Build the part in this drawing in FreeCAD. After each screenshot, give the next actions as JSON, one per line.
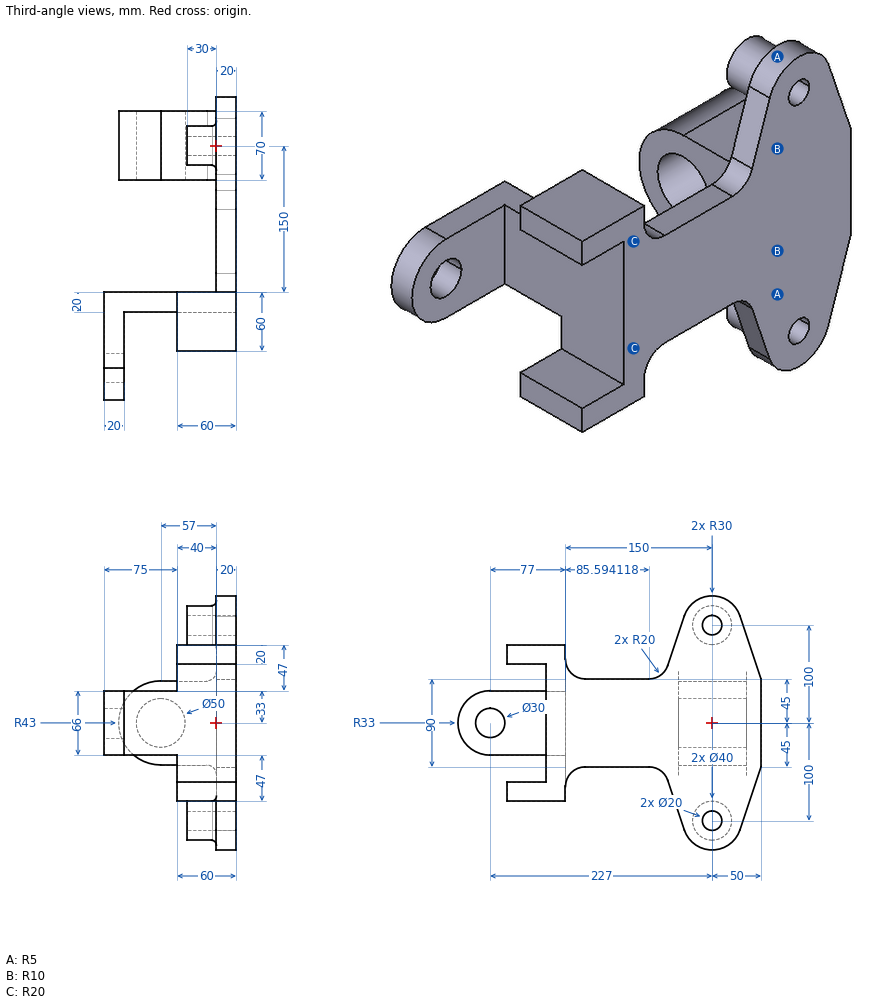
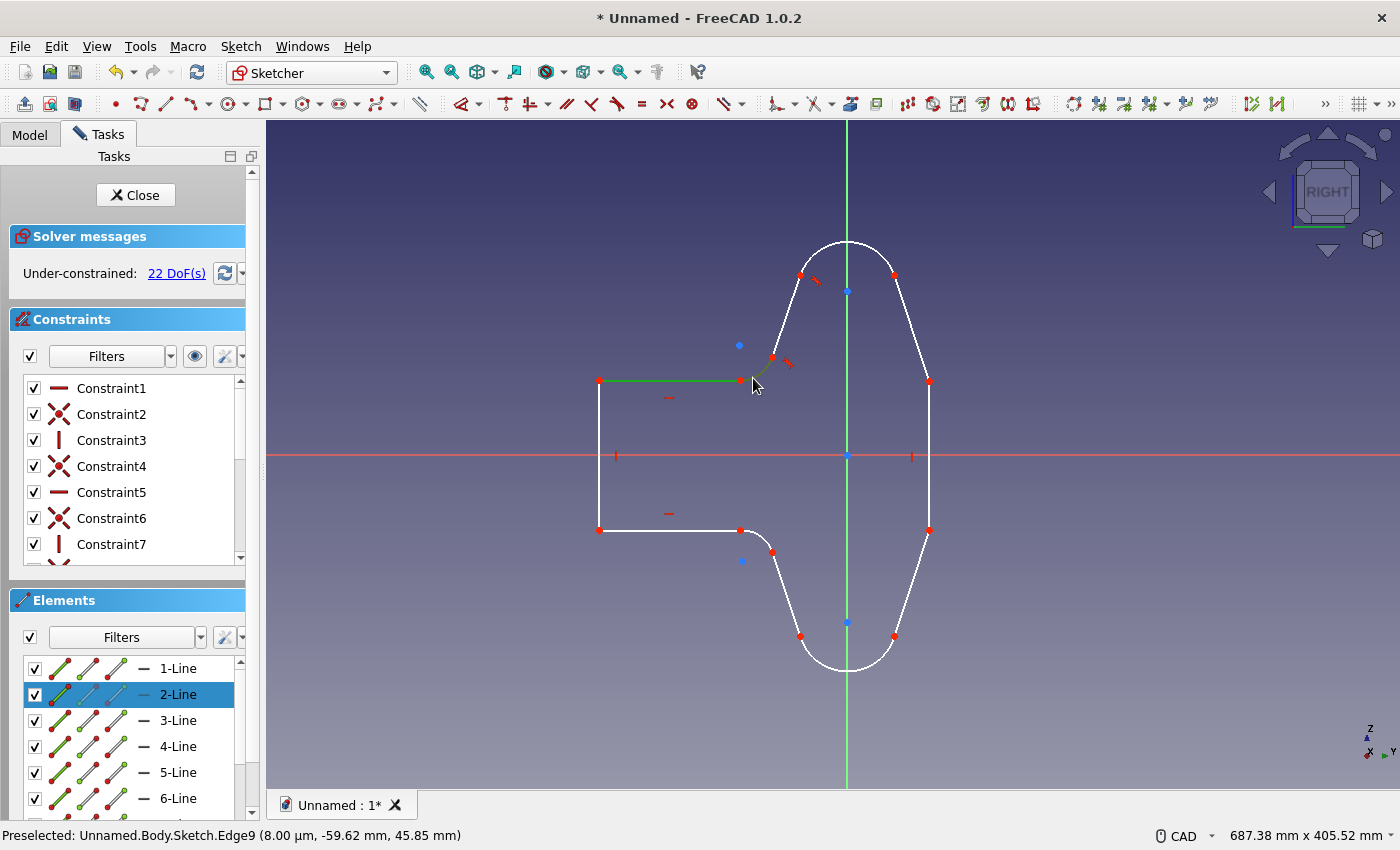
{"action": "left_click", "coordinate": [617, 104]}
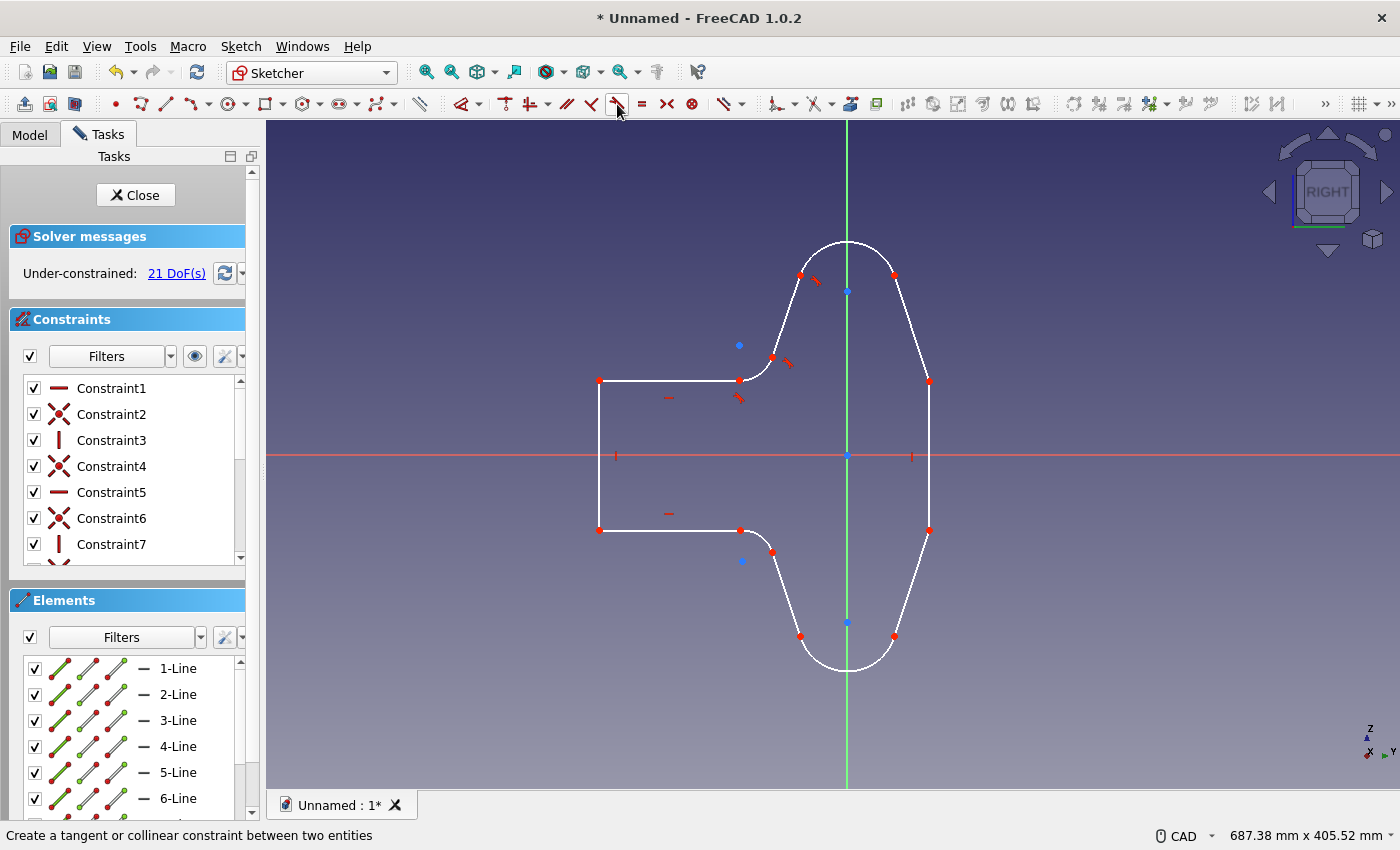
{"action": "left_click", "coordinate": [642, 531]}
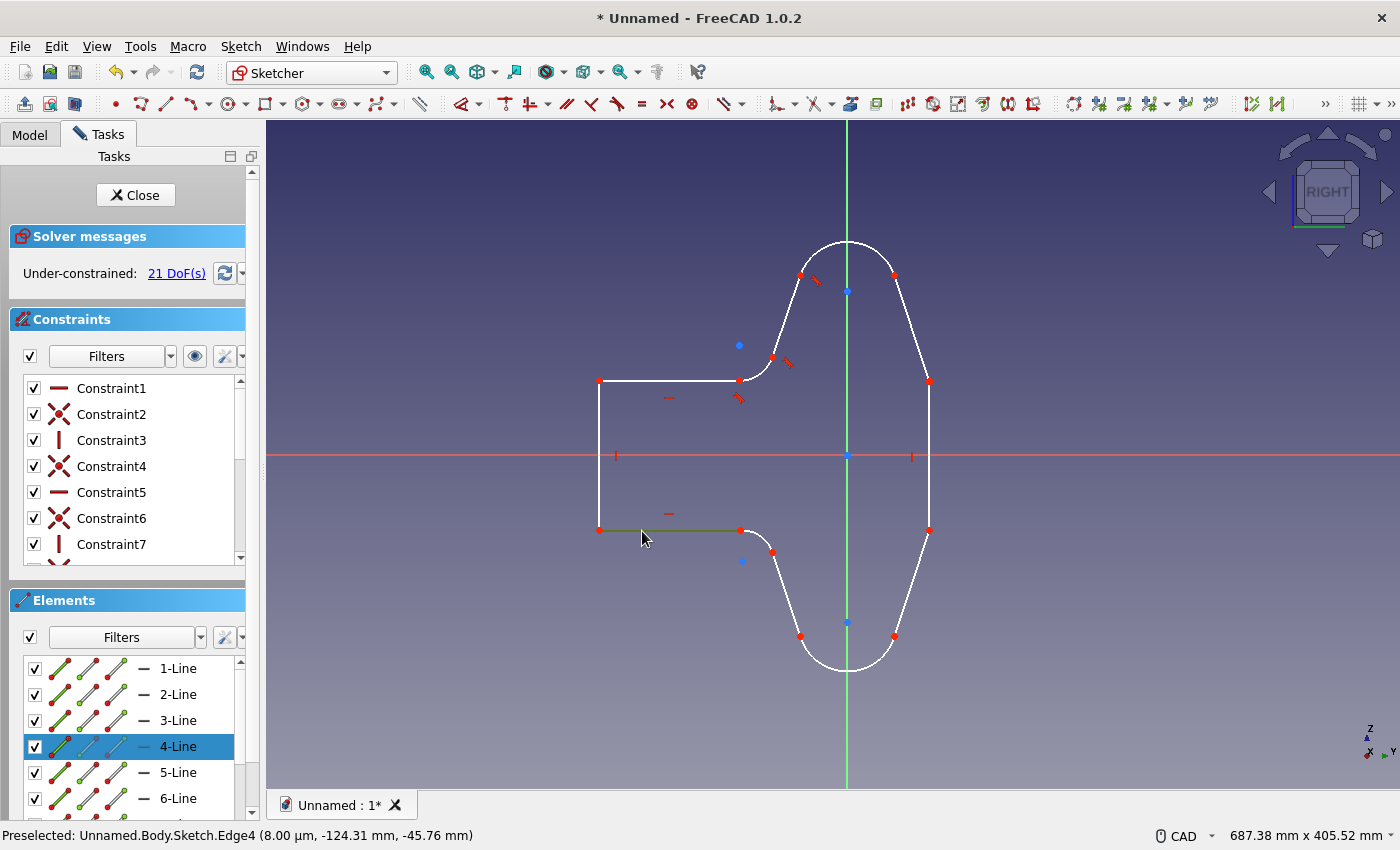
{"action": "left_click", "coordinate": [766, 542]}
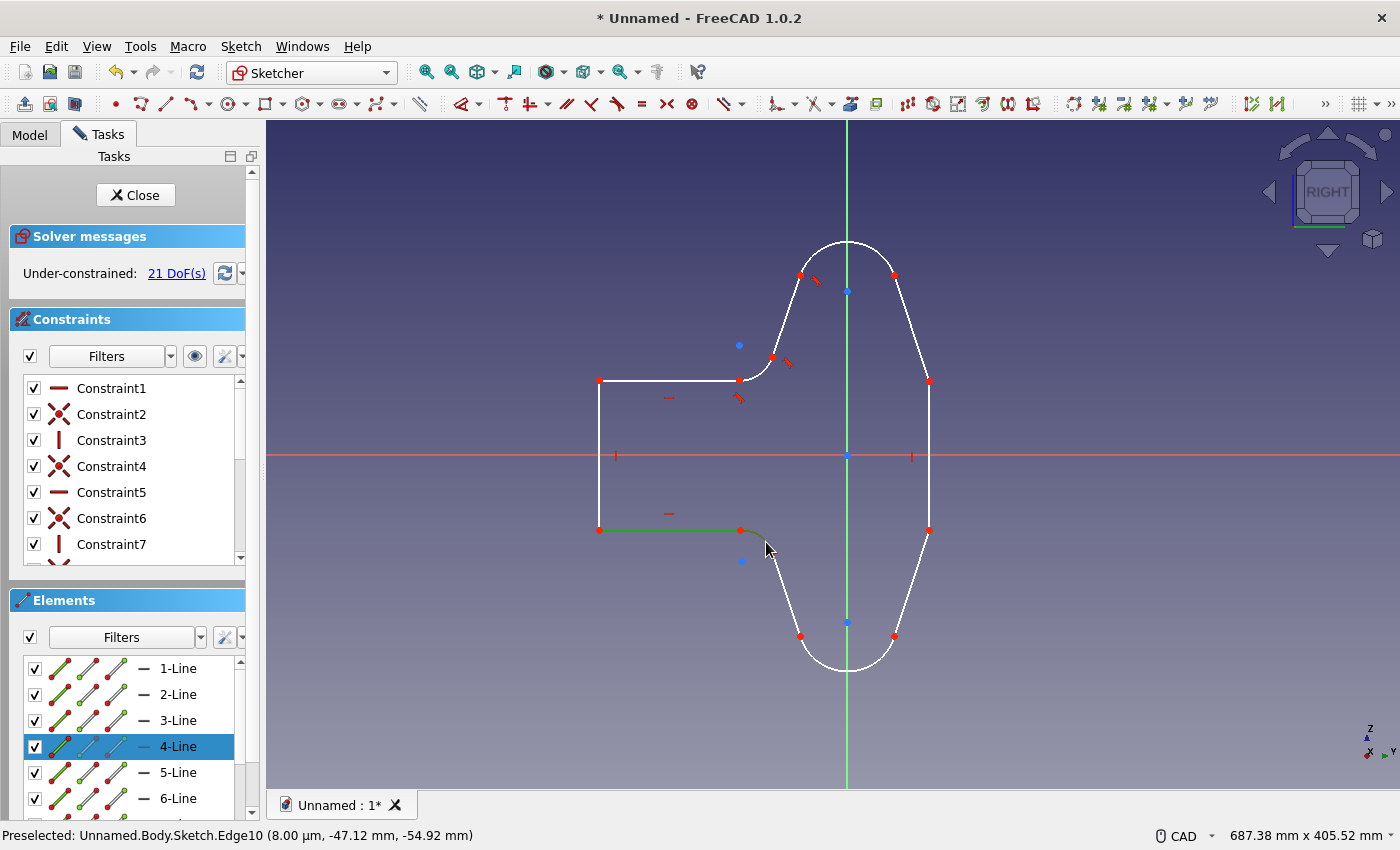
{"action": "left_click", "coordinate": [617, 104]}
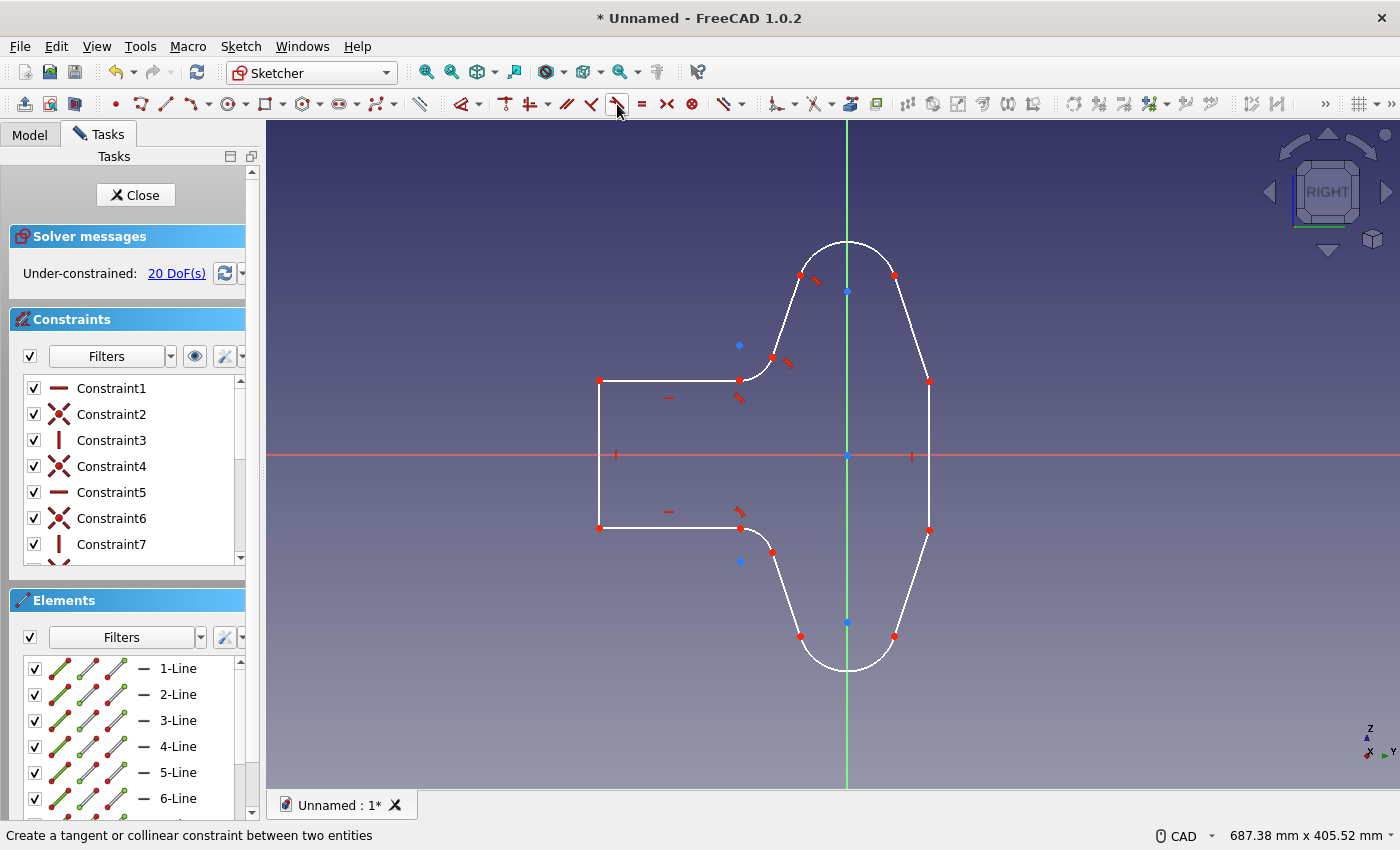
{"action": "left_click", "coordinate": [781, 578]}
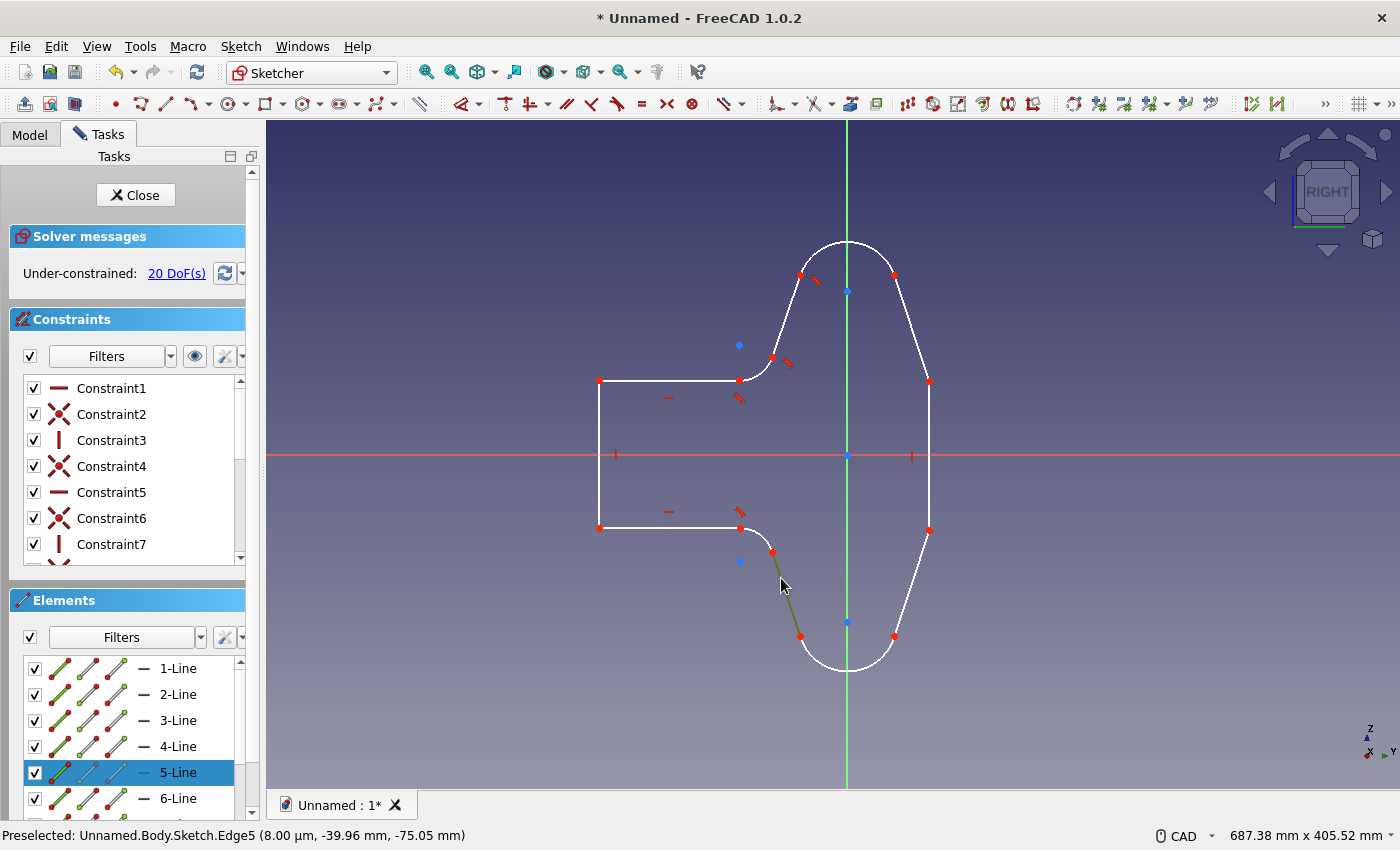
{"action": "left_click", "coordinate": [767, 541]}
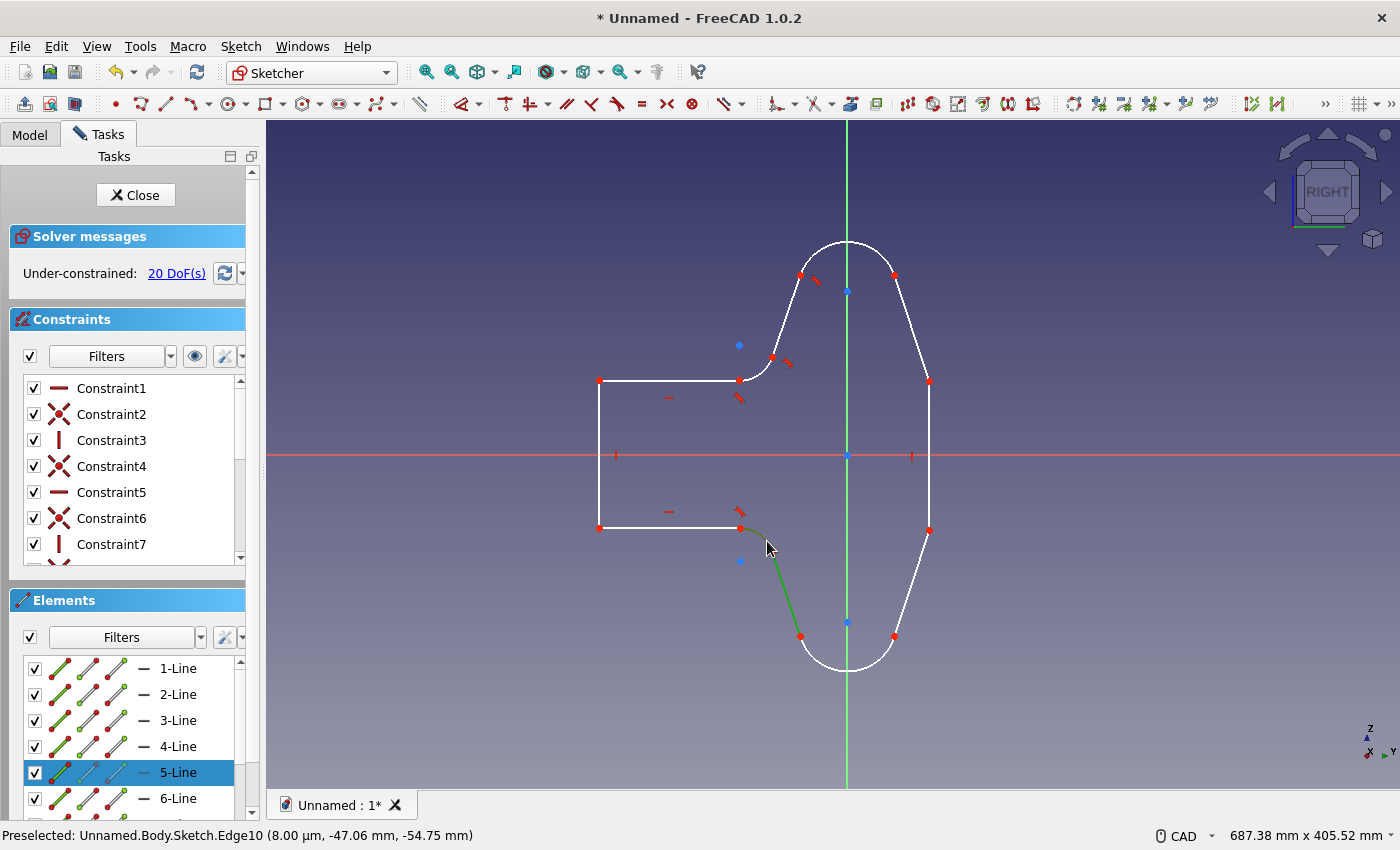
{"action": "left_click", "coordinate": [617, 104]}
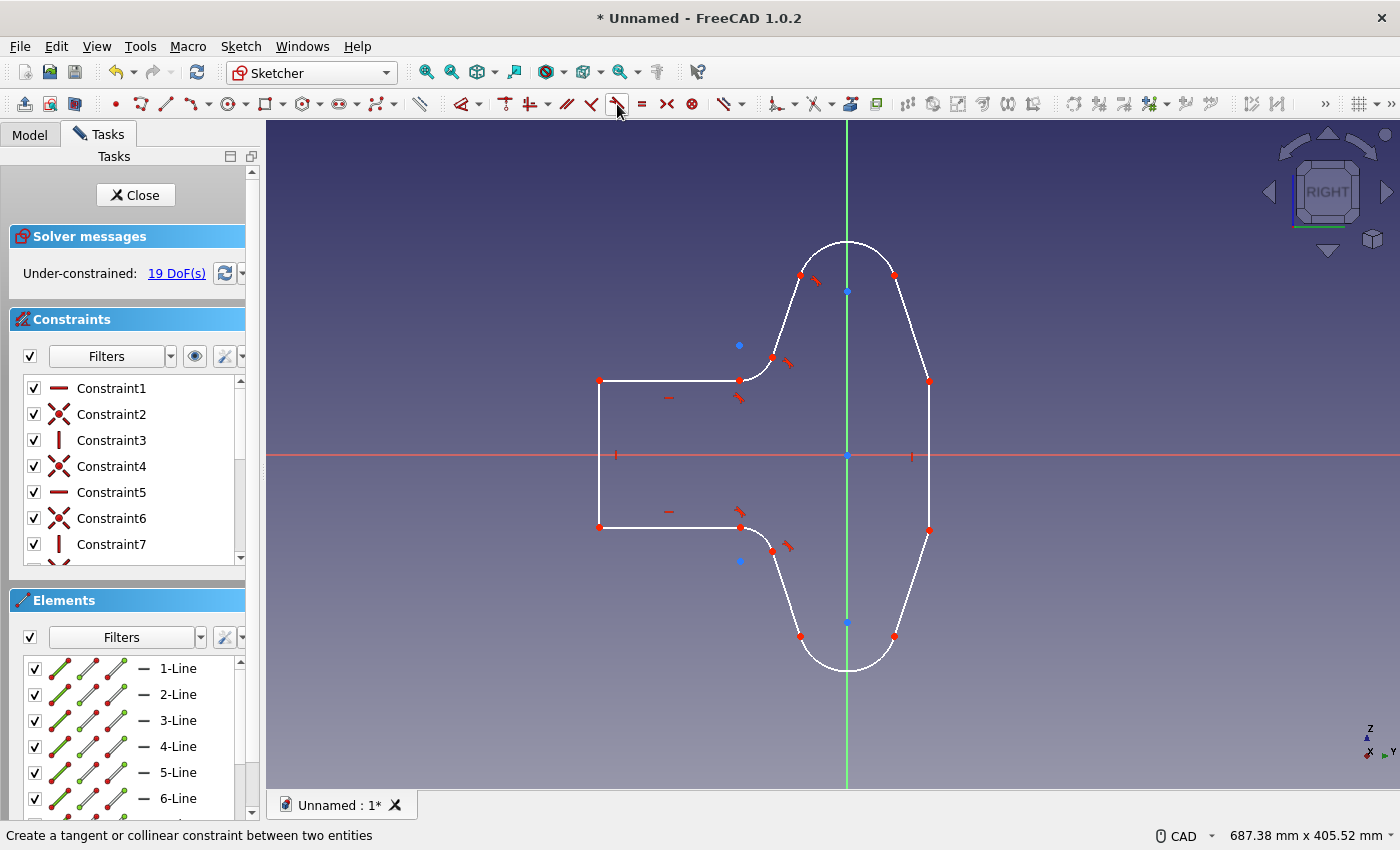
{"action": "left_click", "coordinate": [781, 577]}